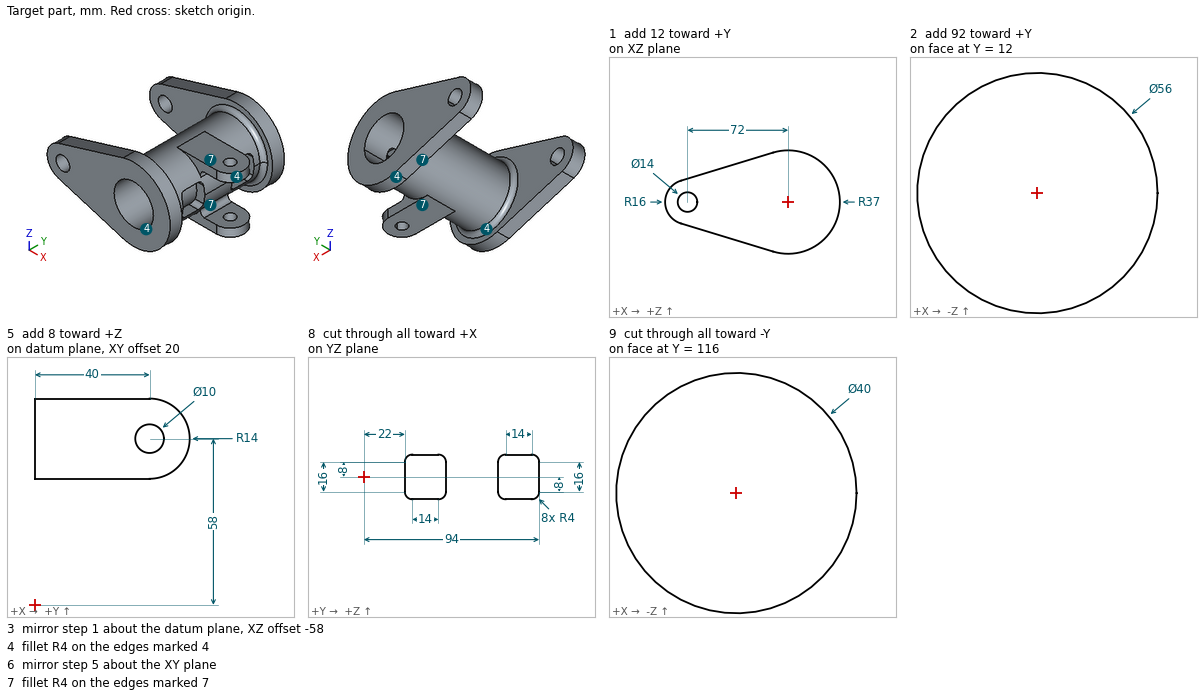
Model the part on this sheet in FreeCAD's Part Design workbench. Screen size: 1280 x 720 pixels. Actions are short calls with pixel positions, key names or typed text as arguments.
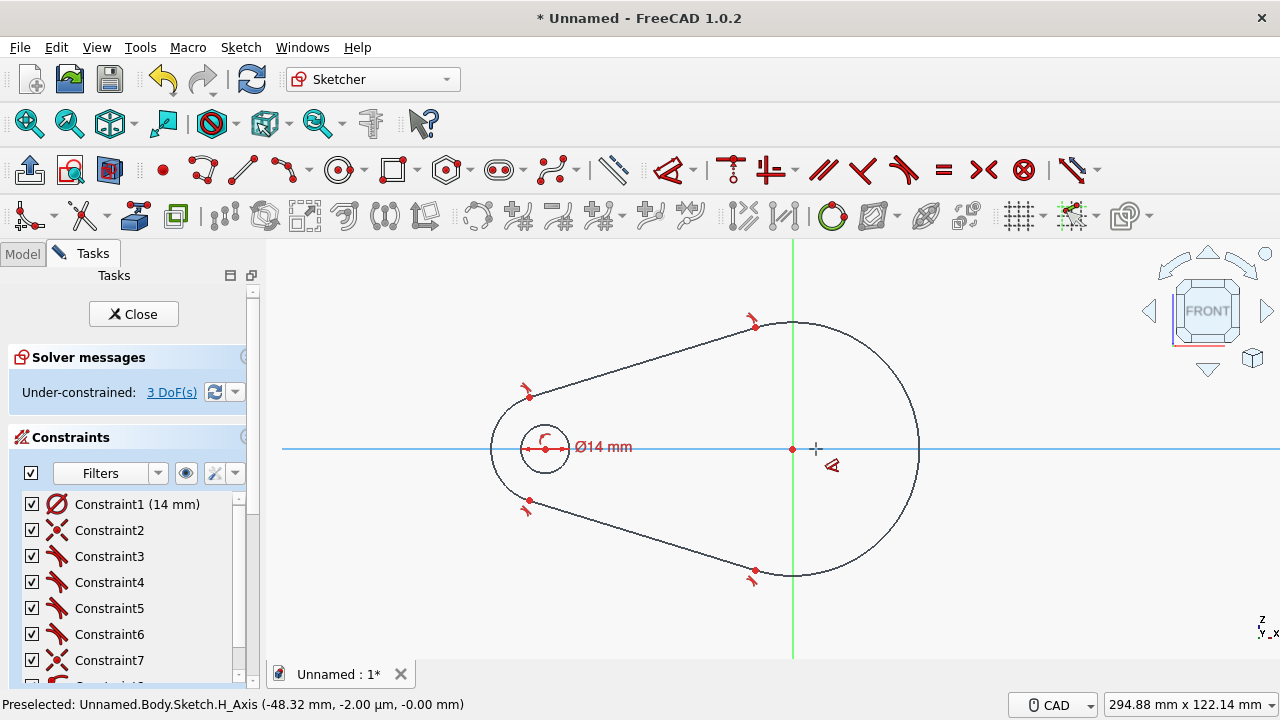
click(498, 423)
click(470, 407)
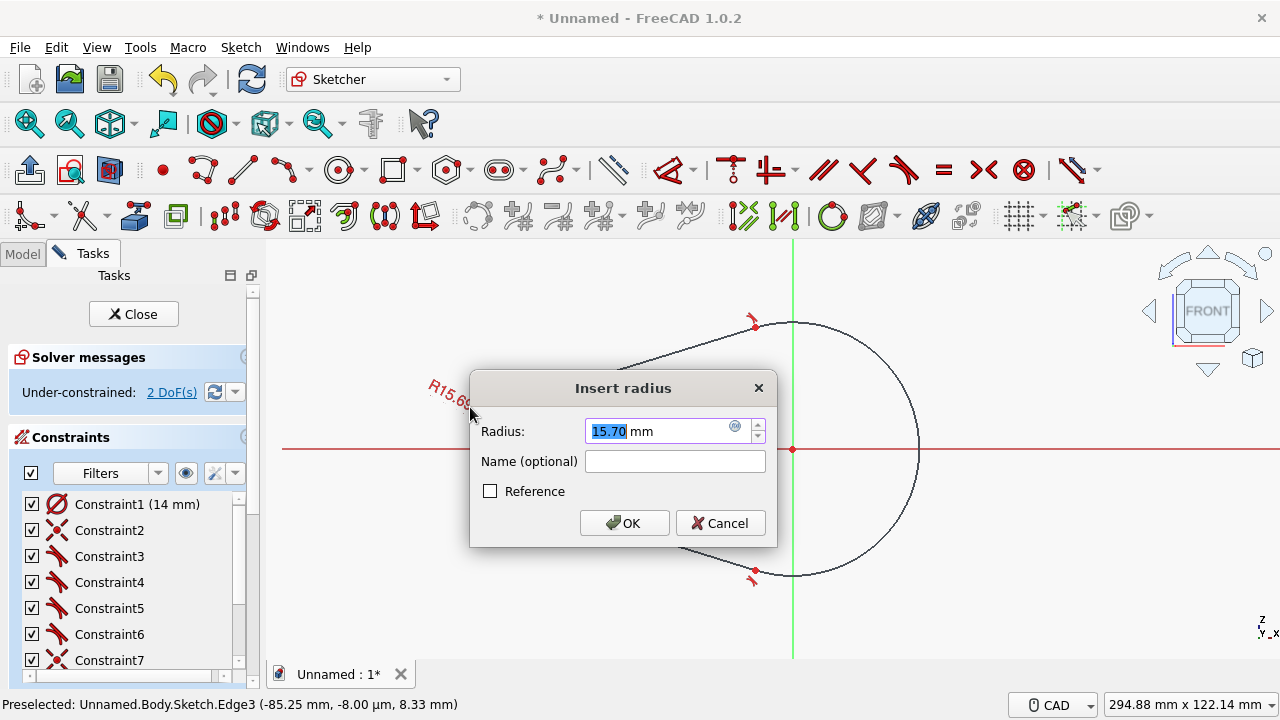
text(16)
key(Return)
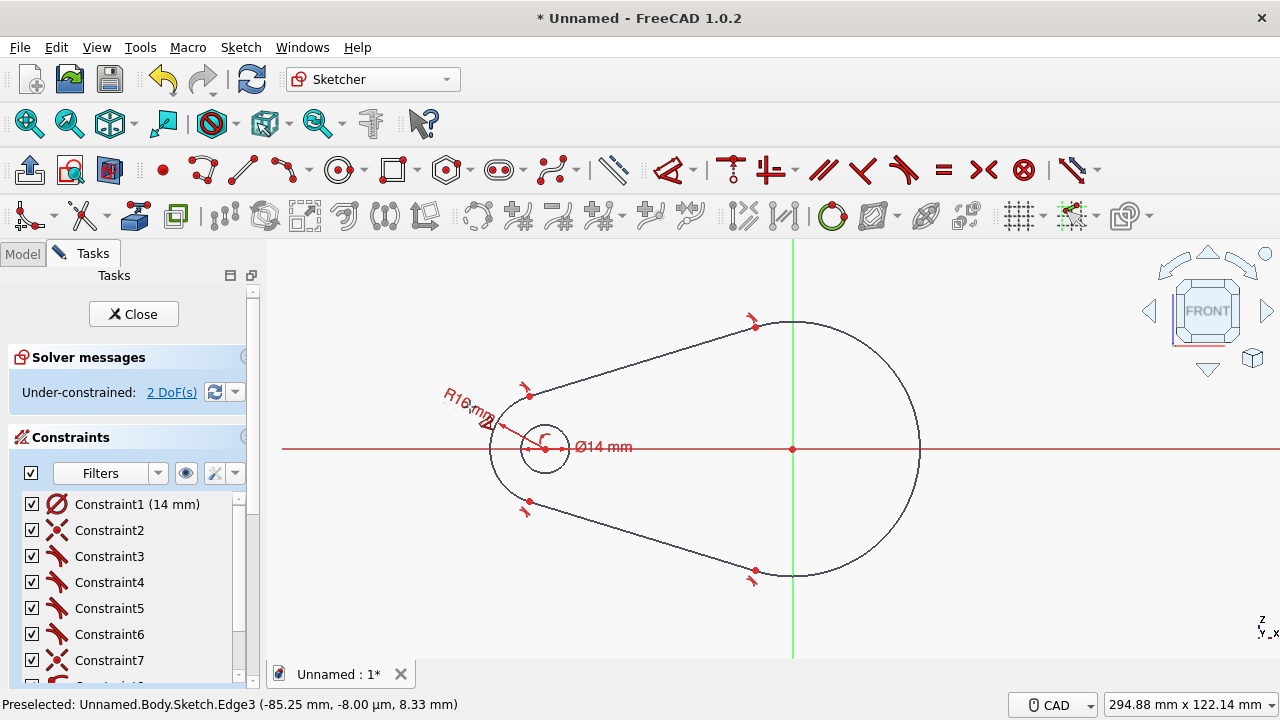
click(886, 536)
click(909, 558)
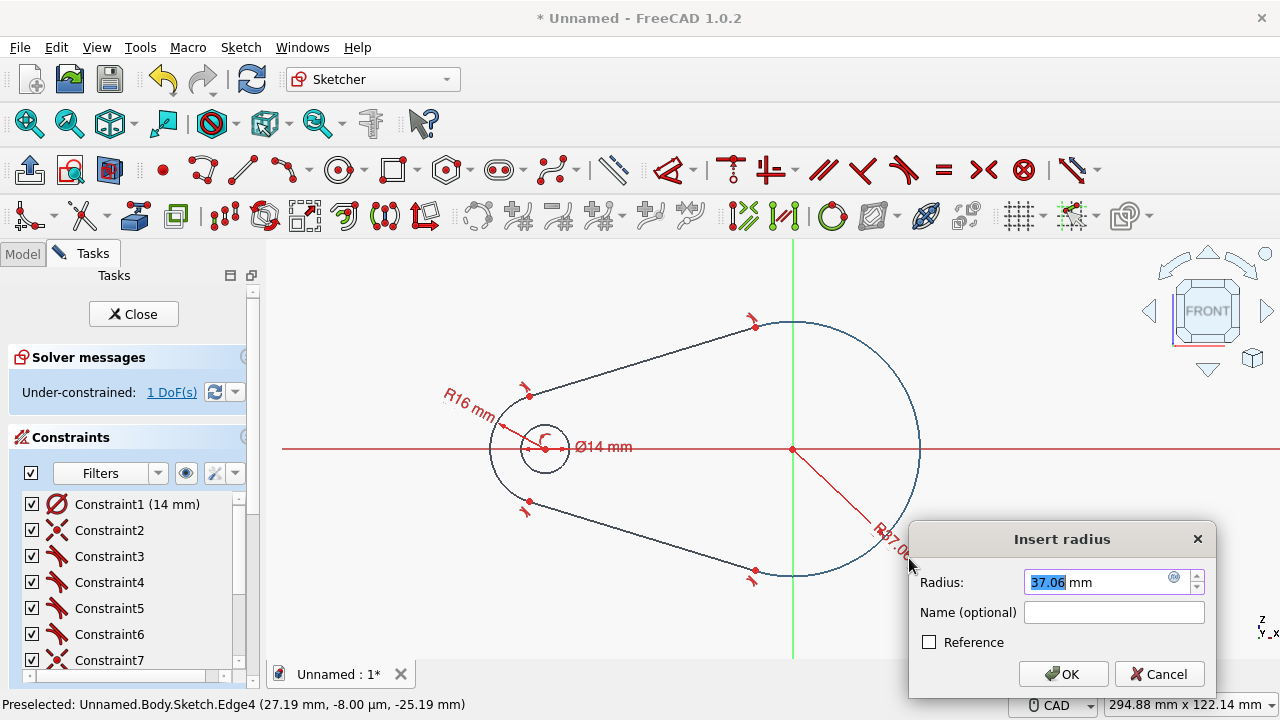
text(37)
key(Return)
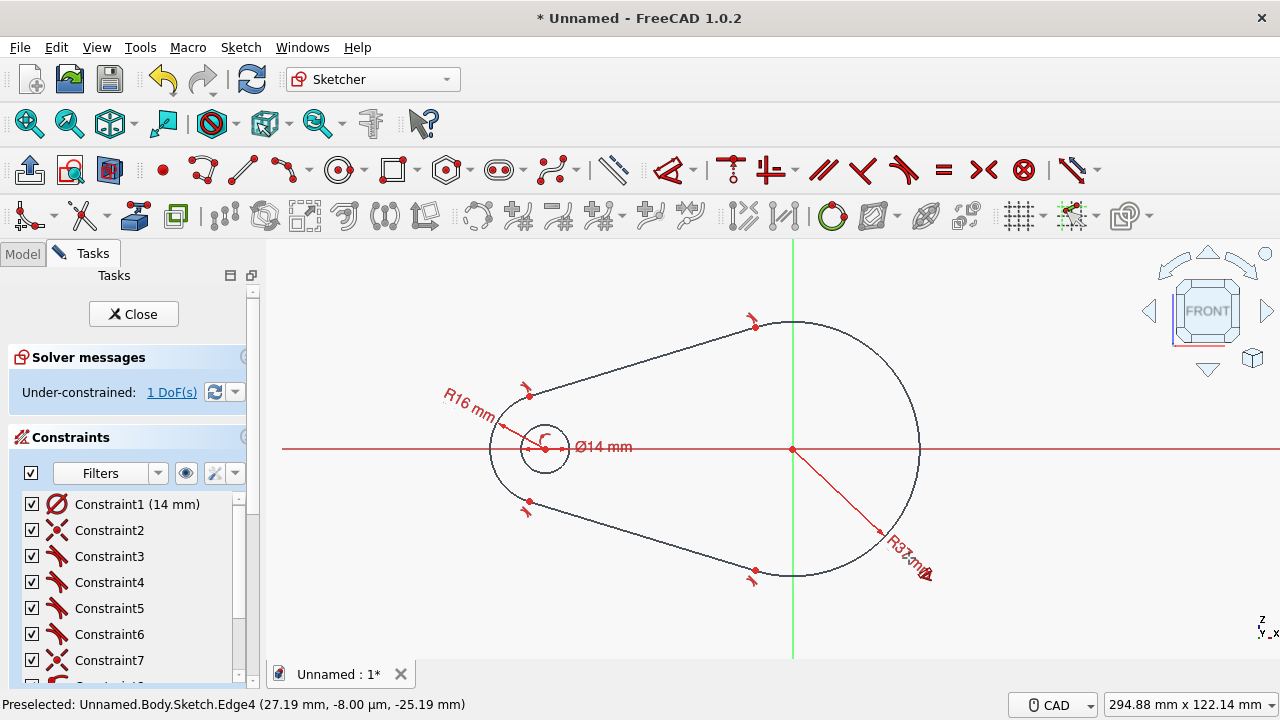
click(545, 449)
click(669, 483)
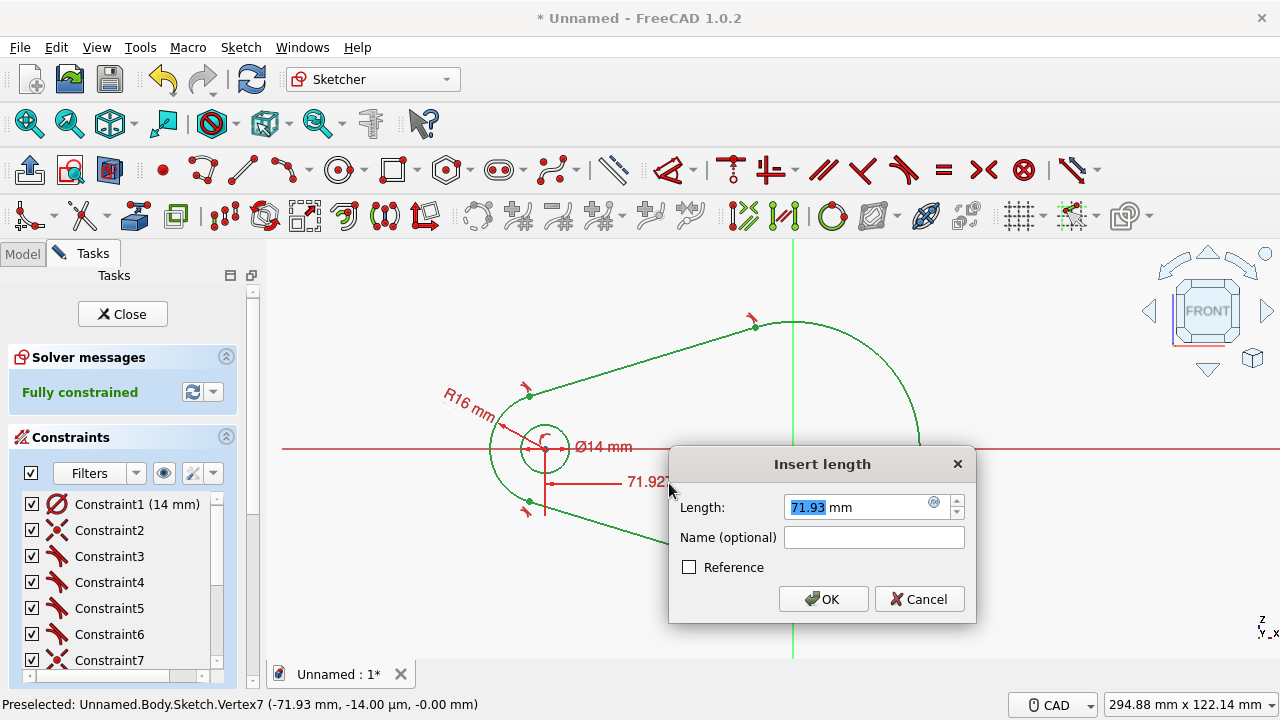
text(72)
key(Return)
key(Escape)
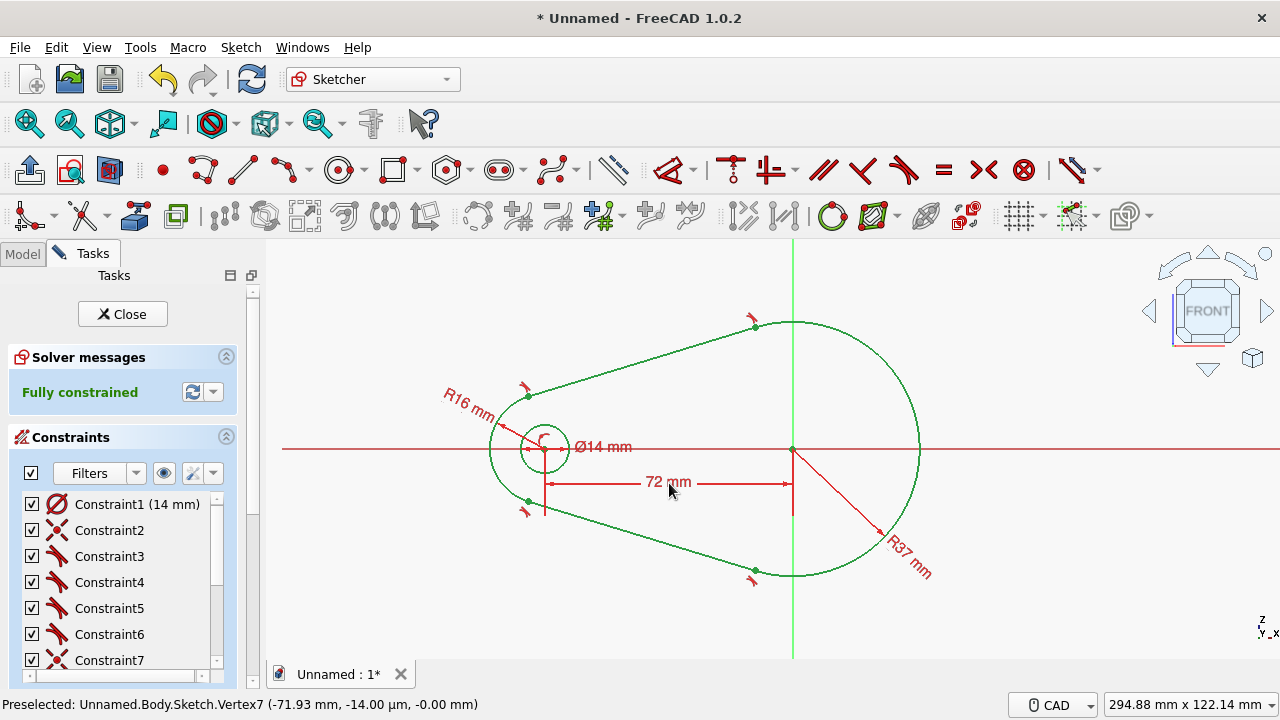
click(123, 314)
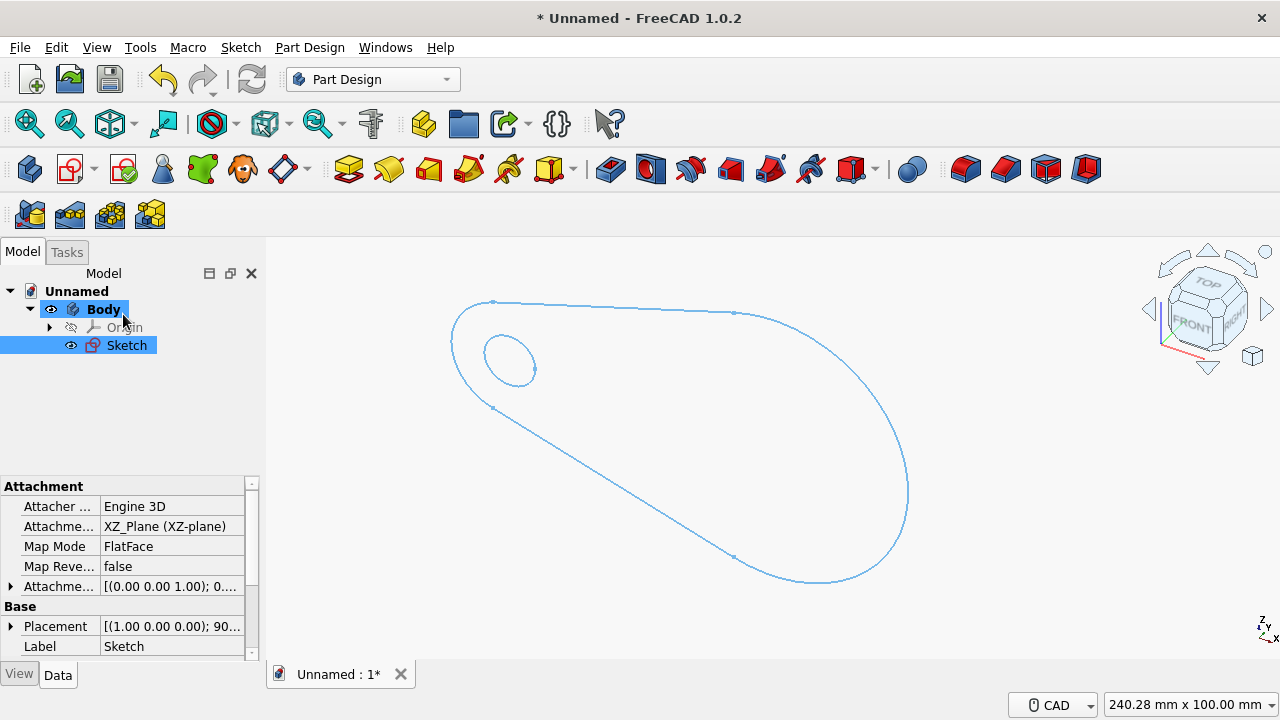
click(350, 170)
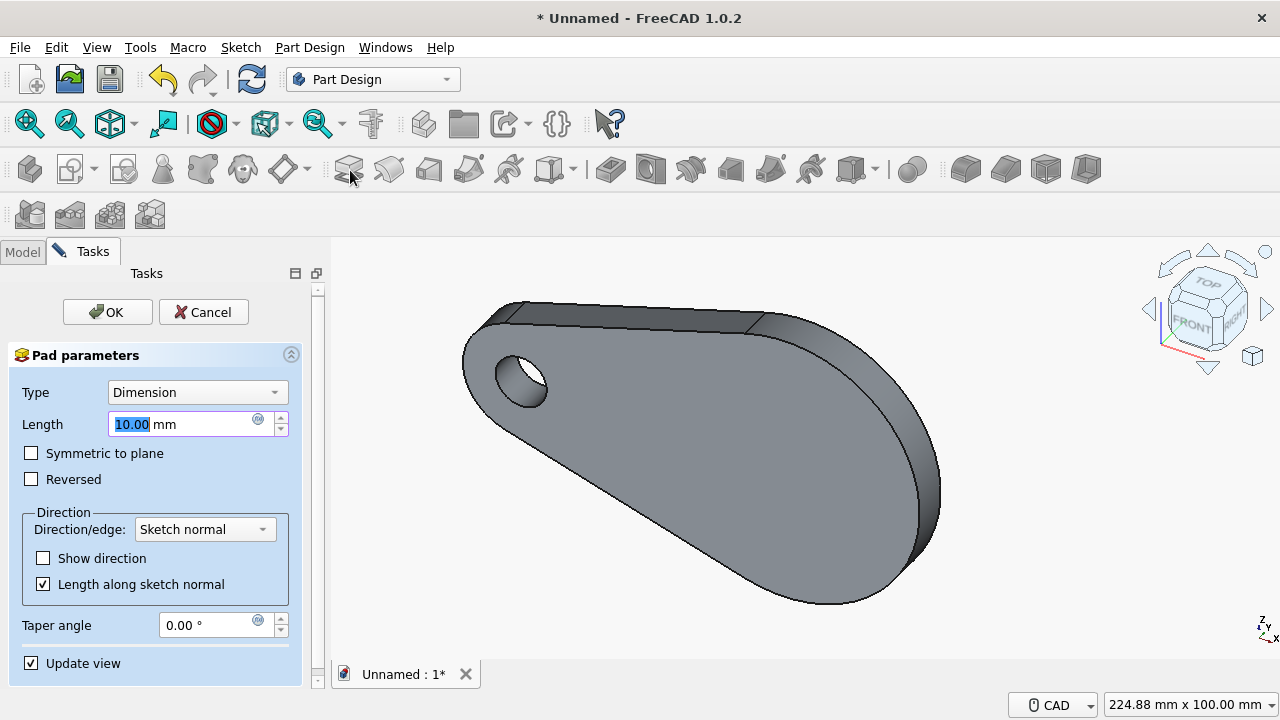
text(12)
key(Tab)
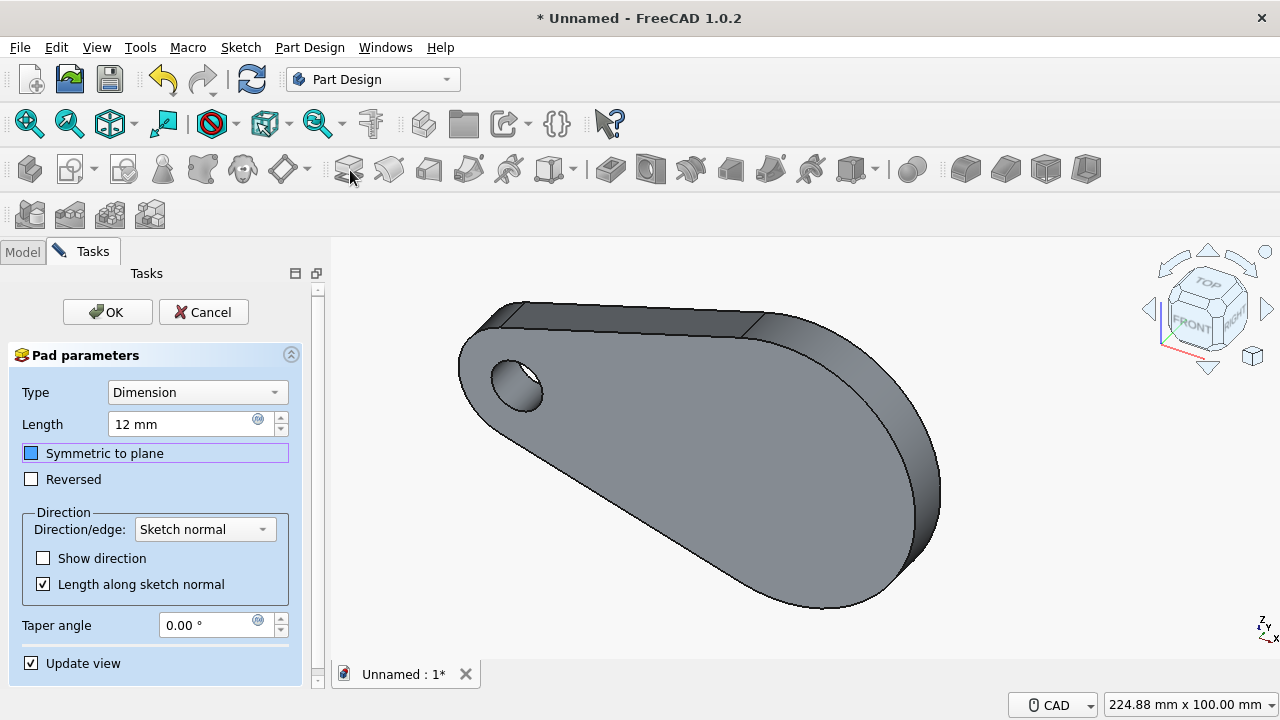
click(30, 479)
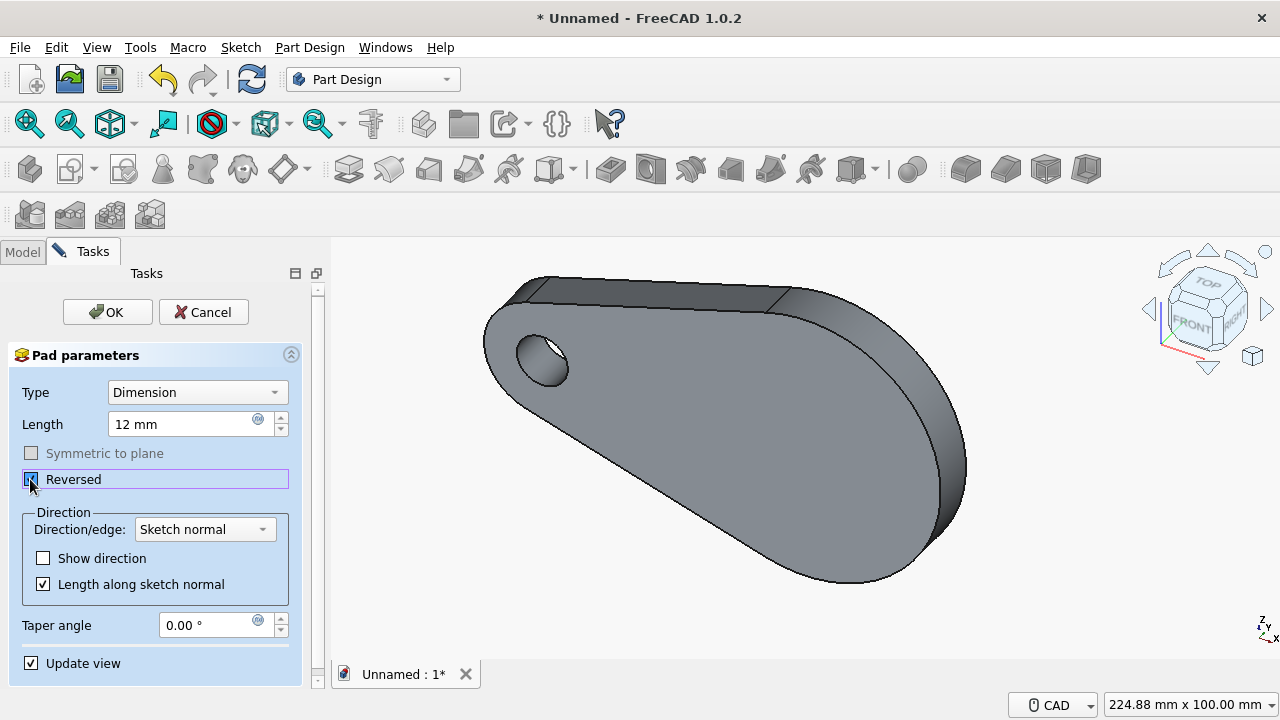
click(108, 312)